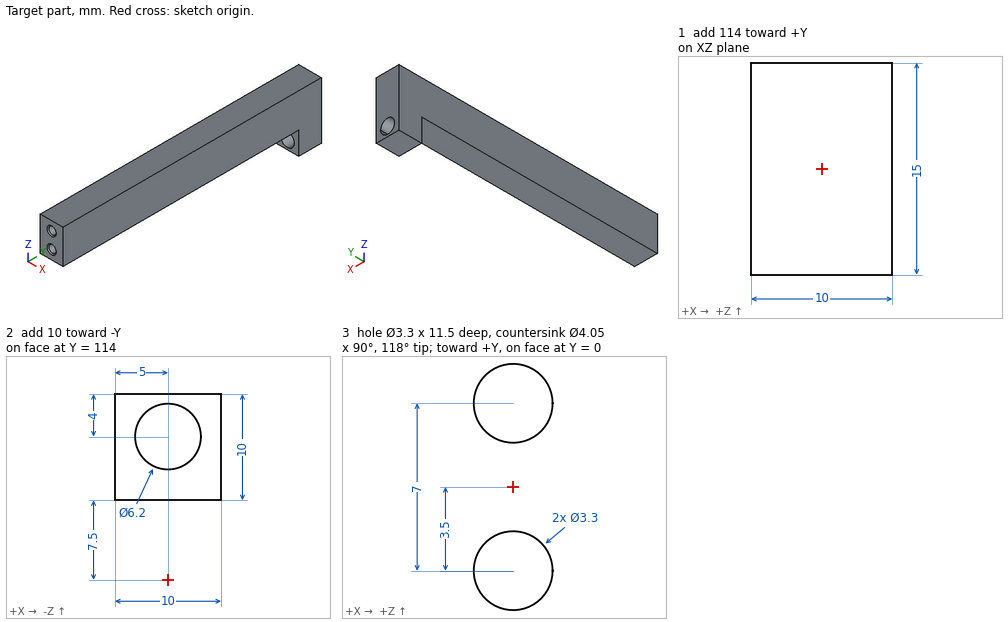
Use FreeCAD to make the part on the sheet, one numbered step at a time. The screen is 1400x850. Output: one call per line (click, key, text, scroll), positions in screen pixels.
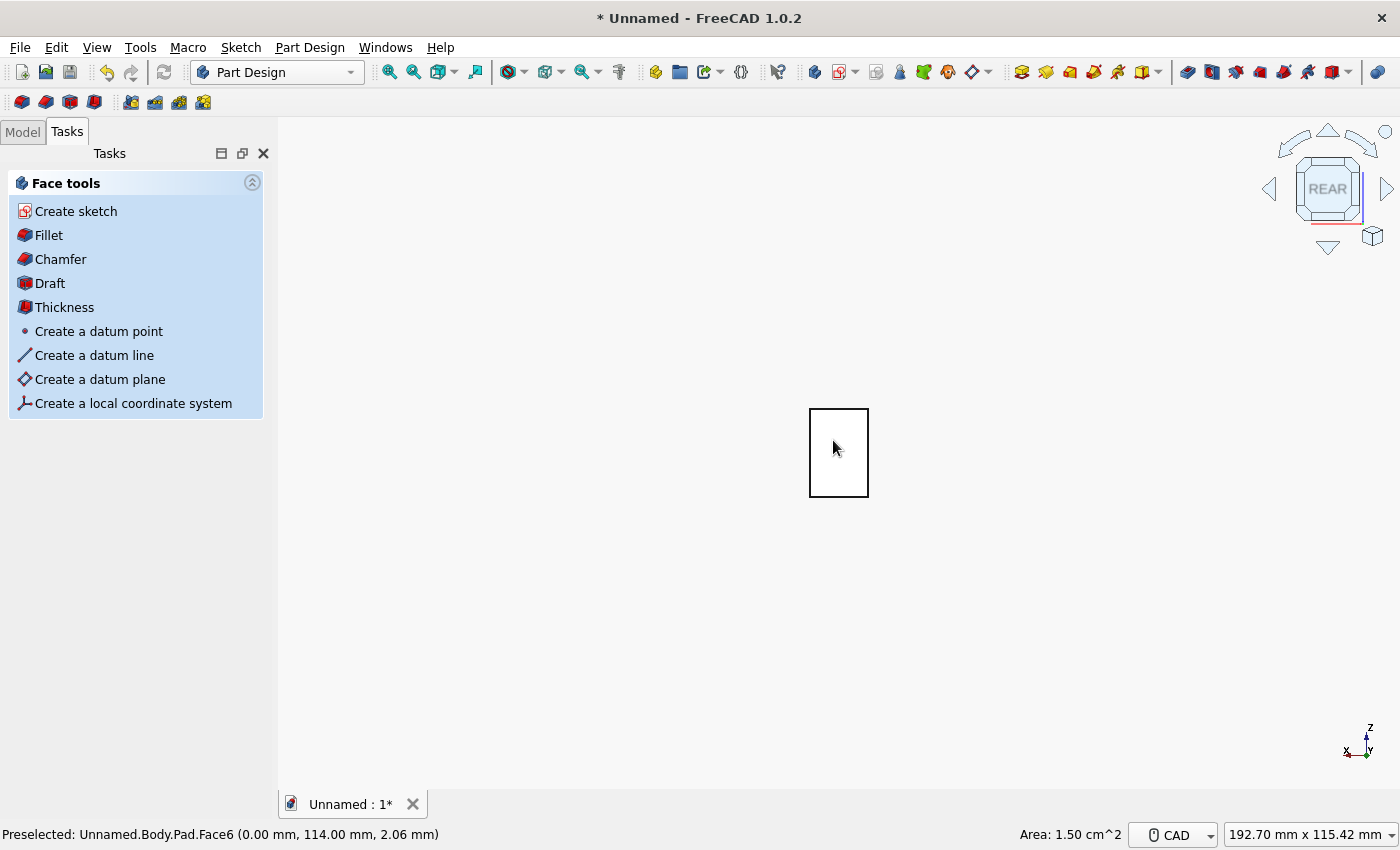
click(840, 72)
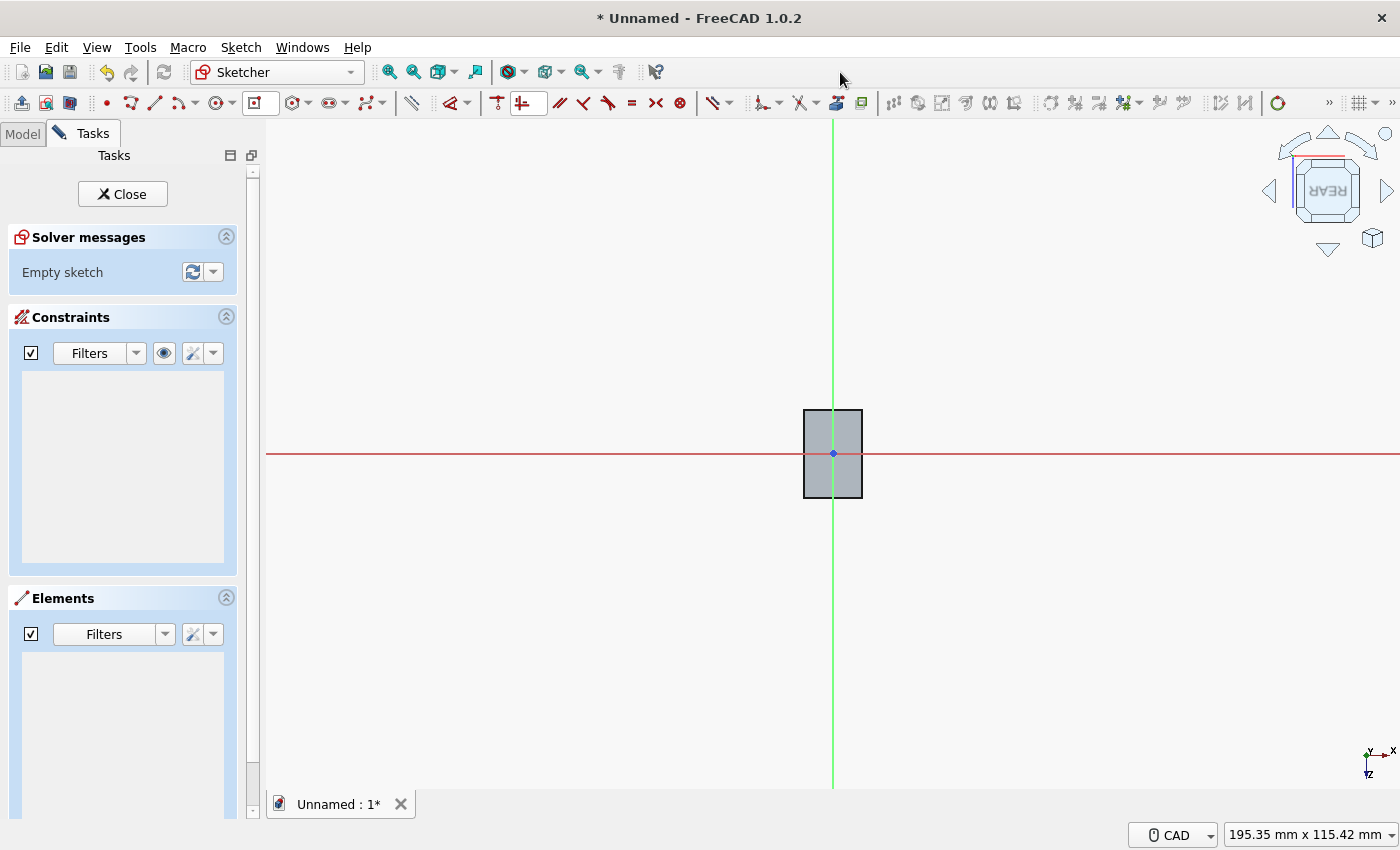
scroll(855, 387, up, 7)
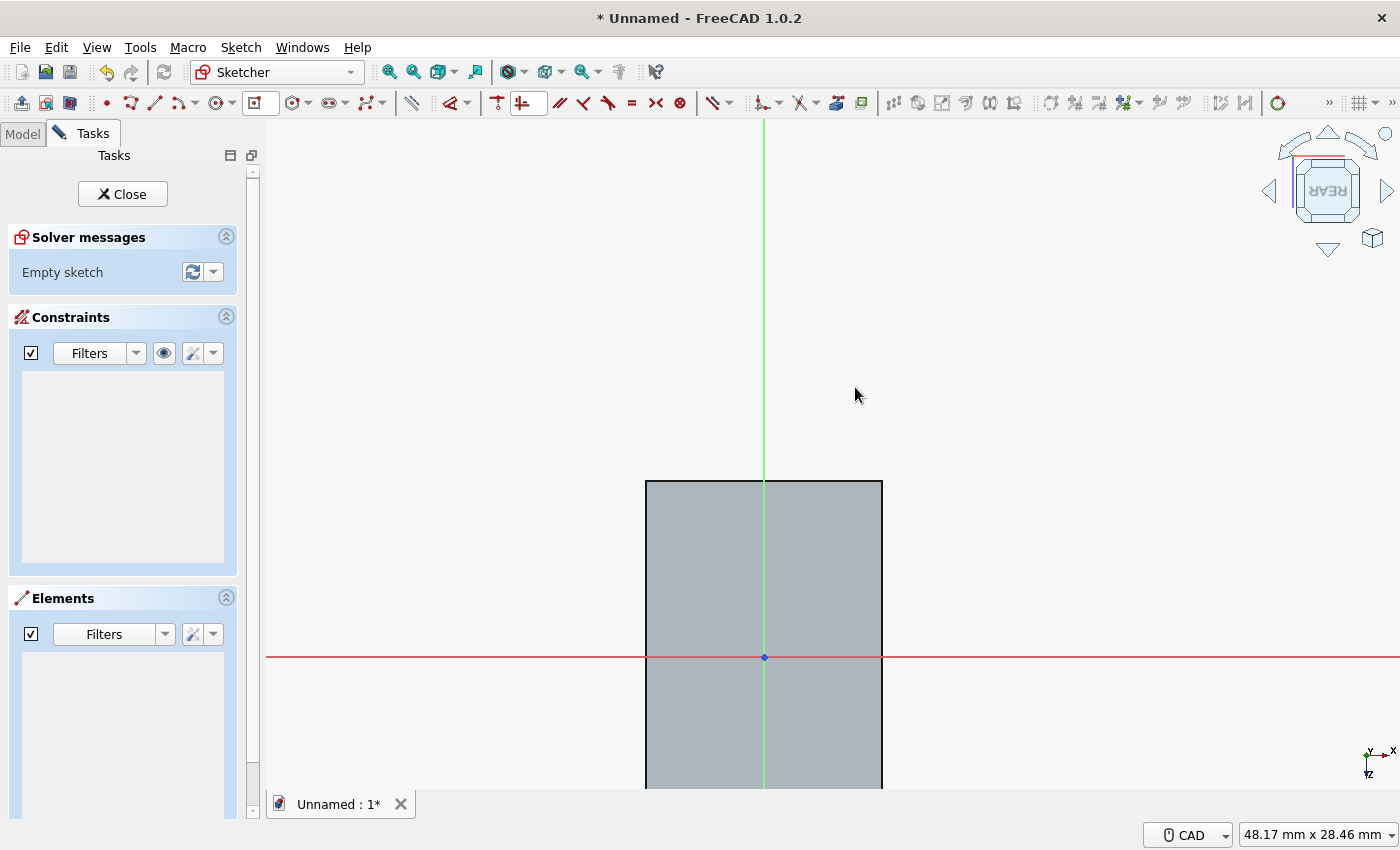
click(274, 104)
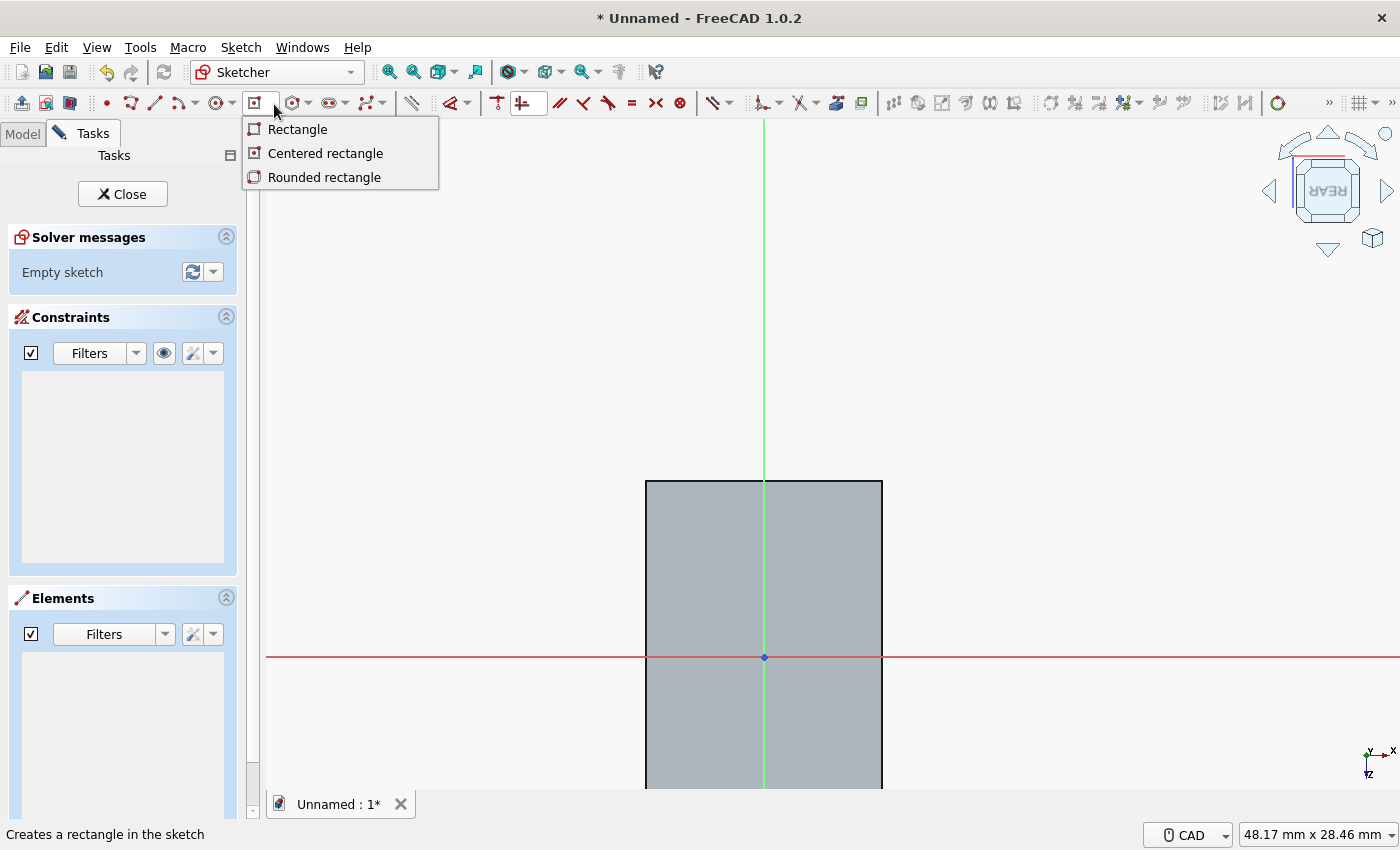
click(340, 129)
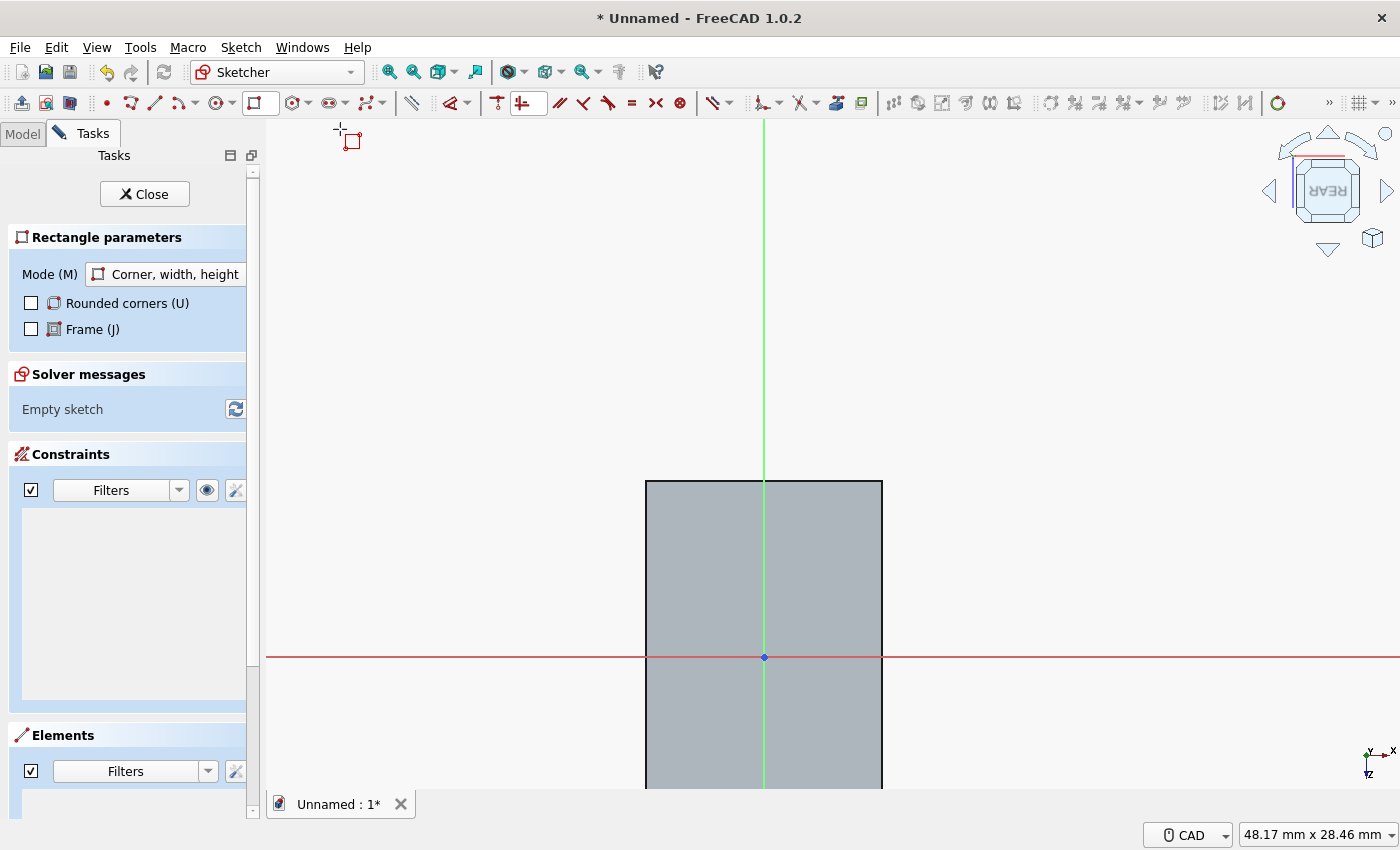
click(646, 246)
move(882, 481)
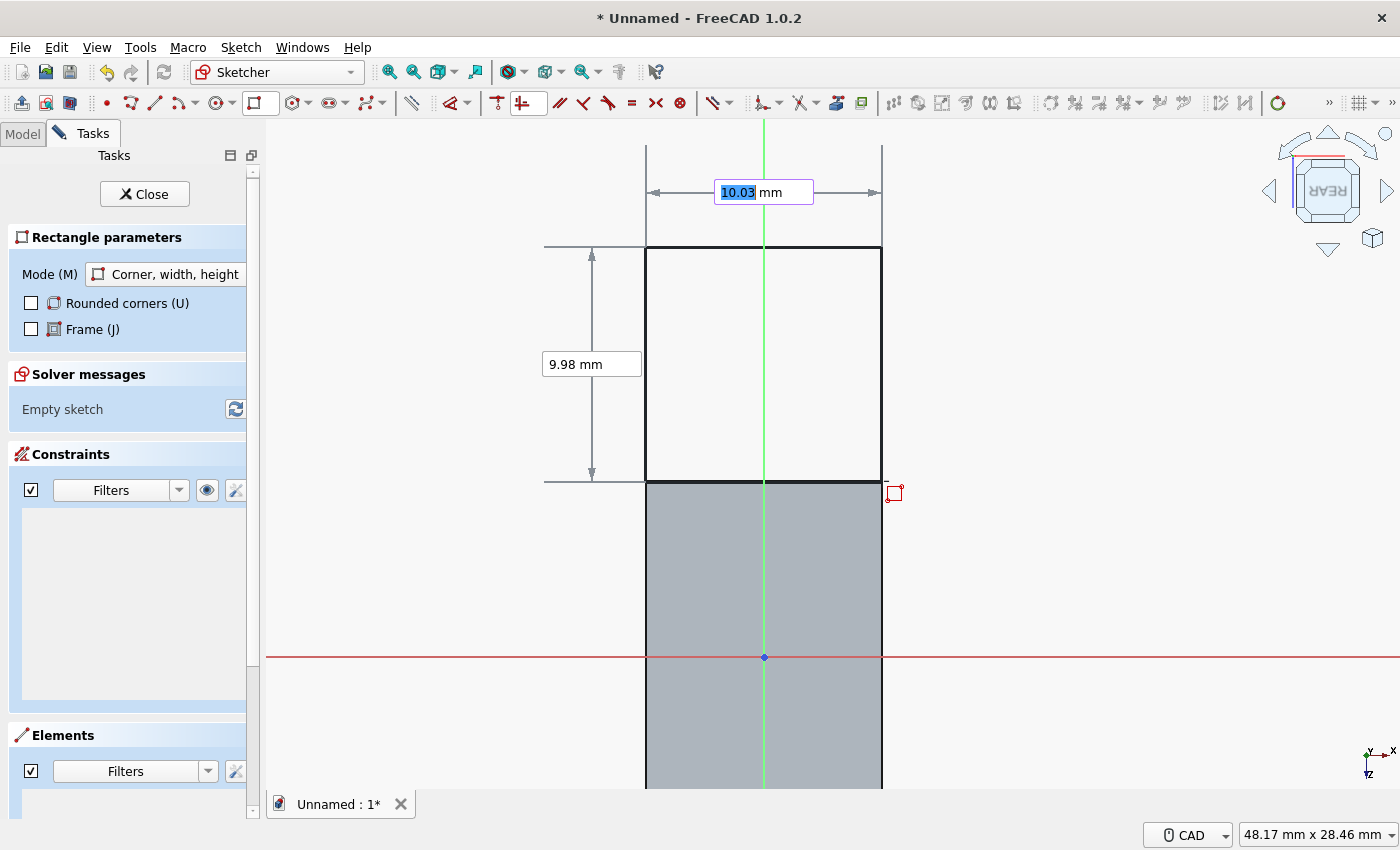
text(10)
key(Tab)
text(10)
key(Return)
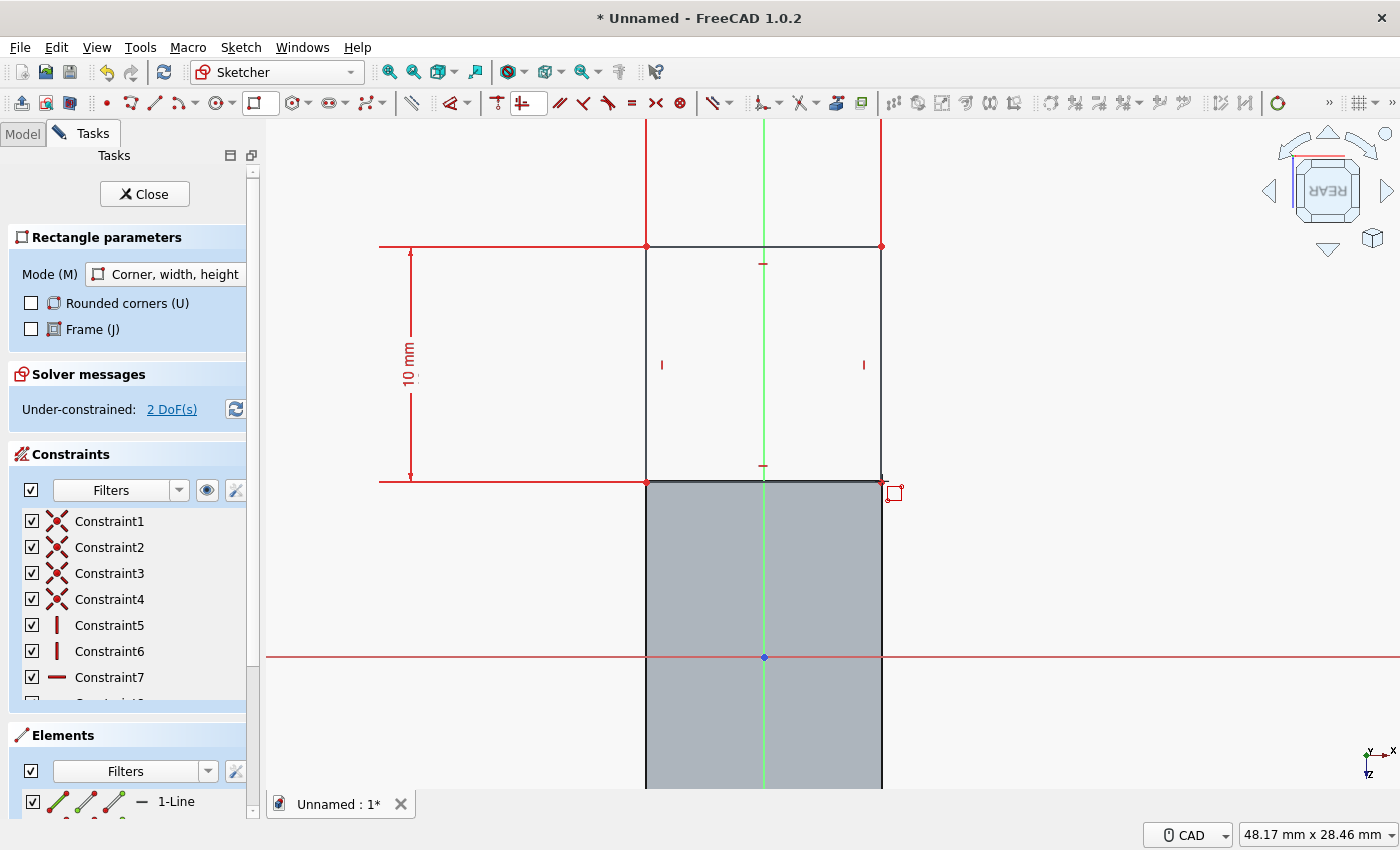
click(216, 104)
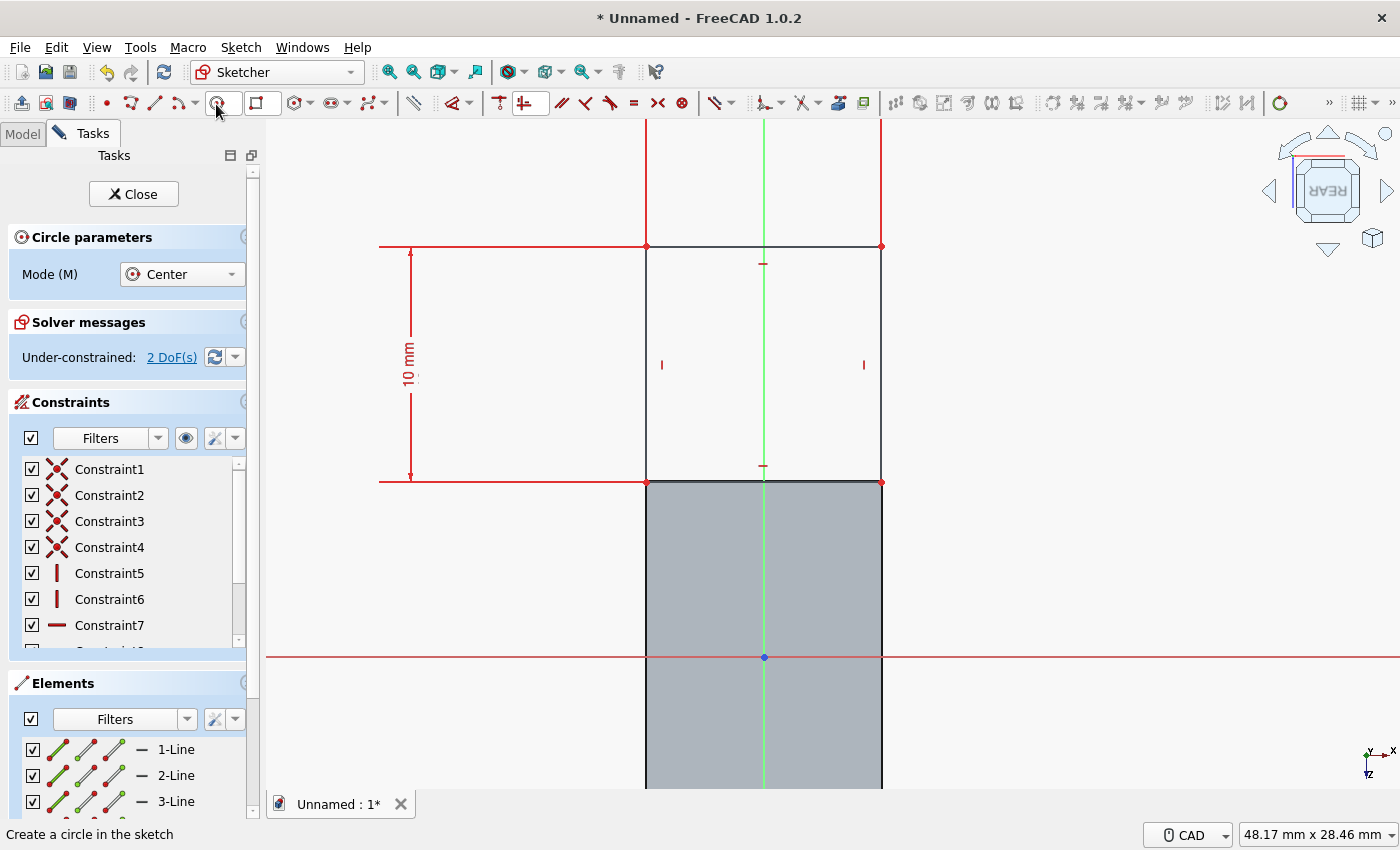
click(764, 340)
move(816, 288)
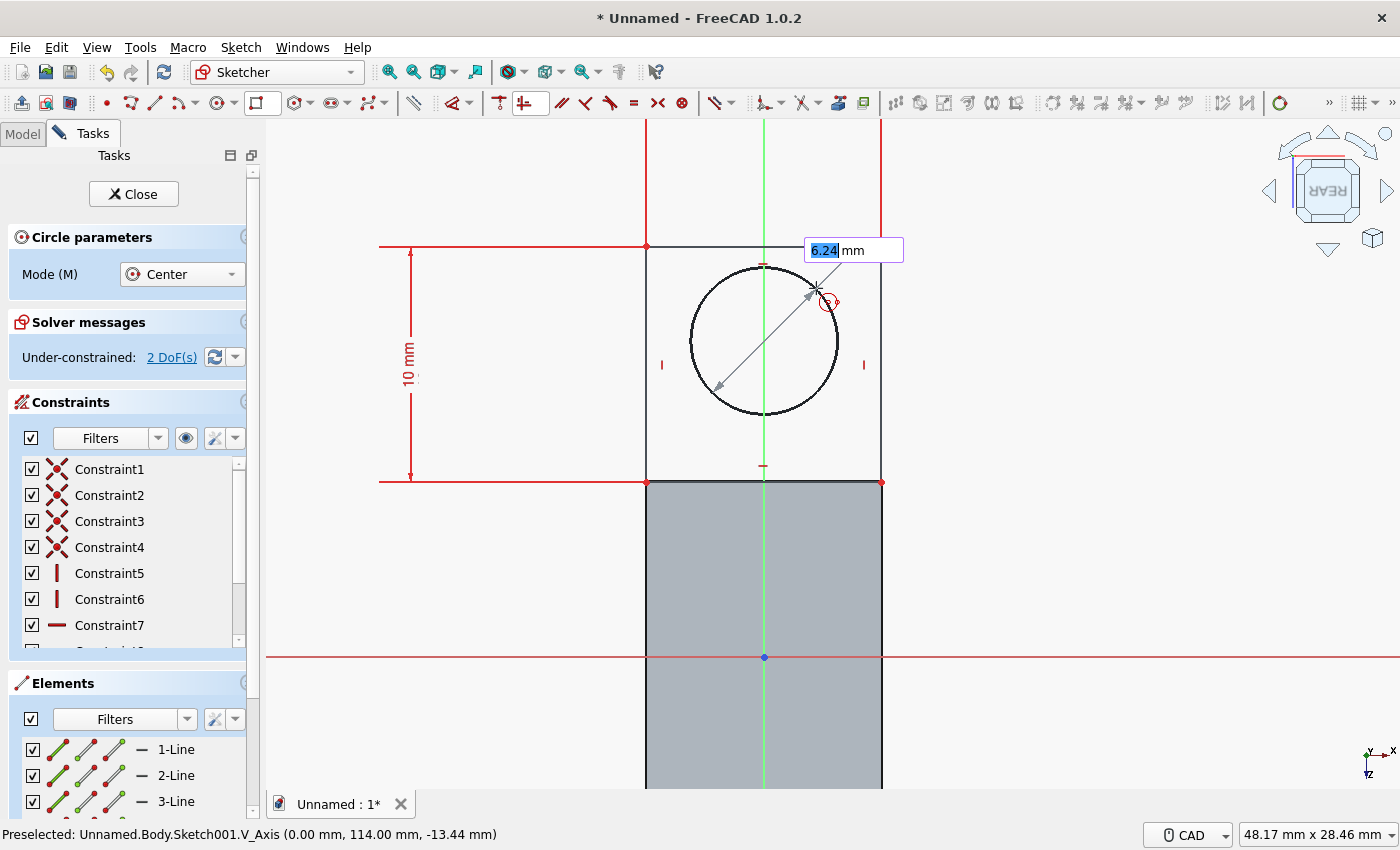
text(6.2)
key(Return)
key(Escape)